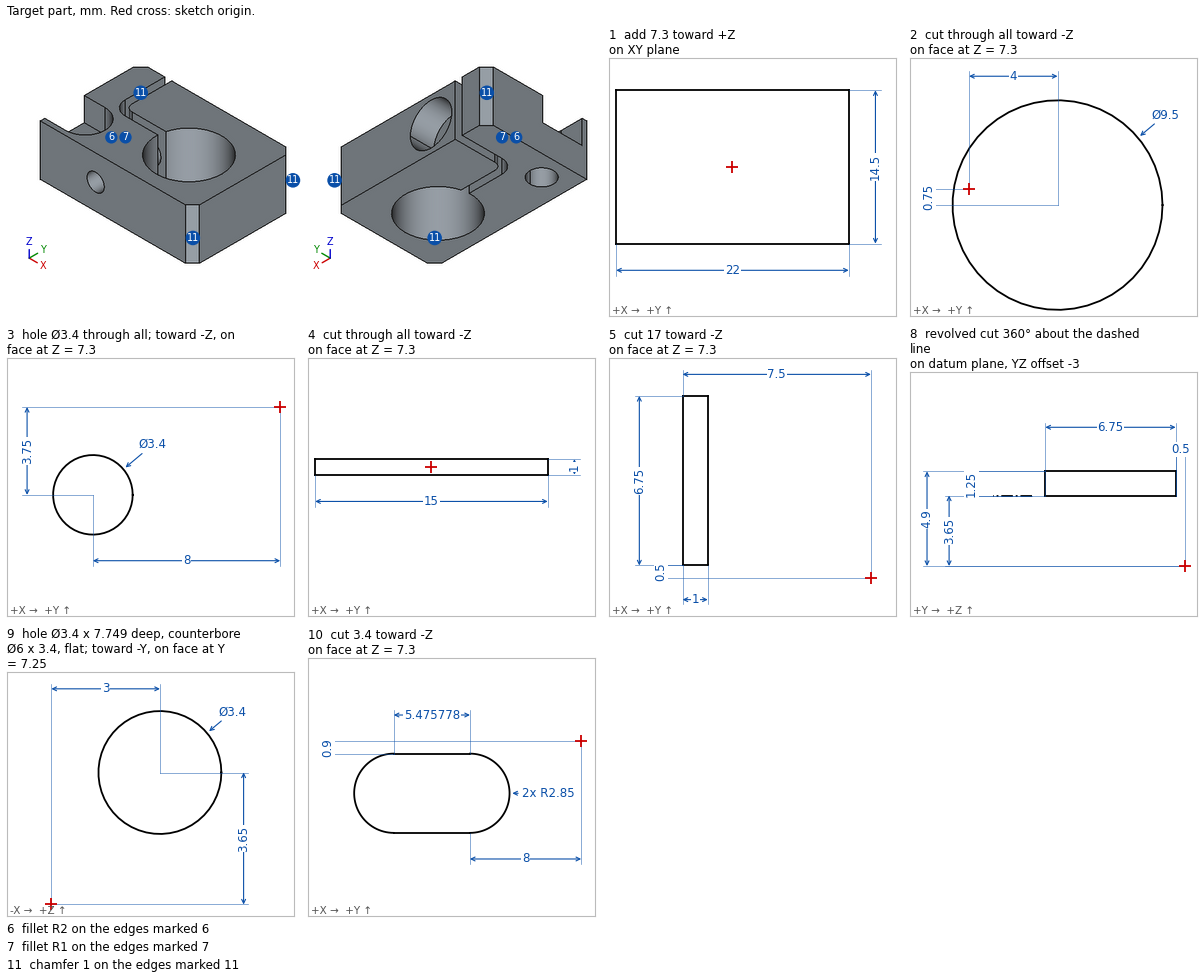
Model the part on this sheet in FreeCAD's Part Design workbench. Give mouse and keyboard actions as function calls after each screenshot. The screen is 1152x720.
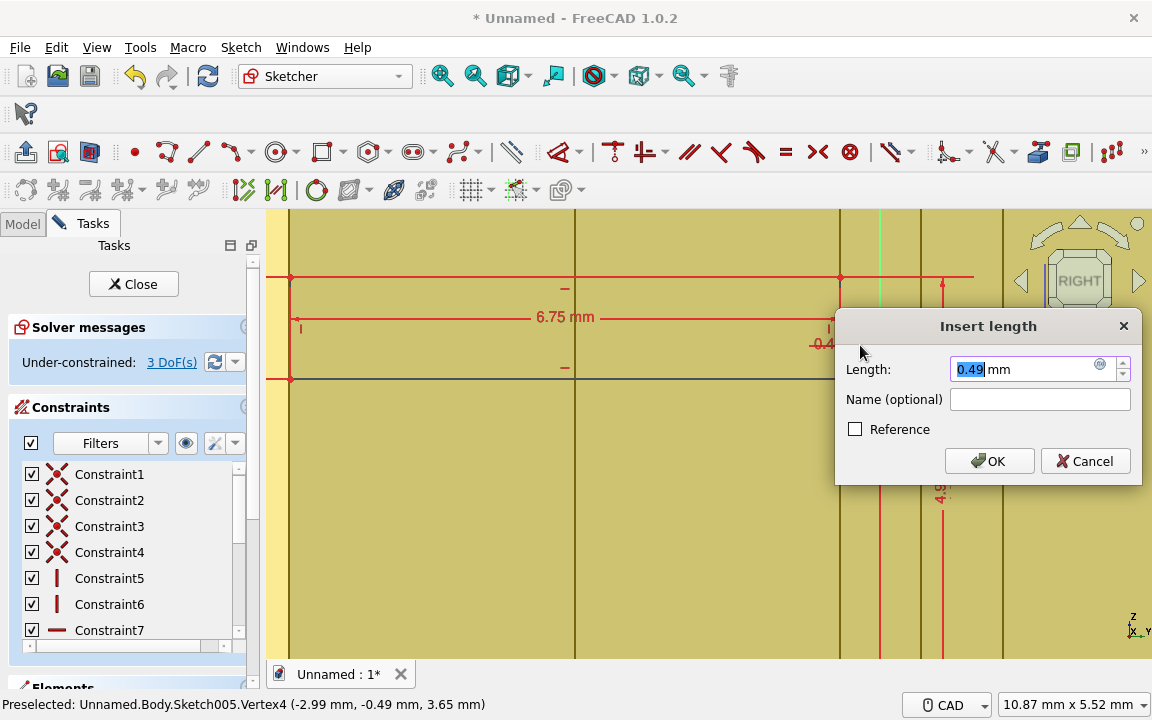
text(0.5)
key(Return)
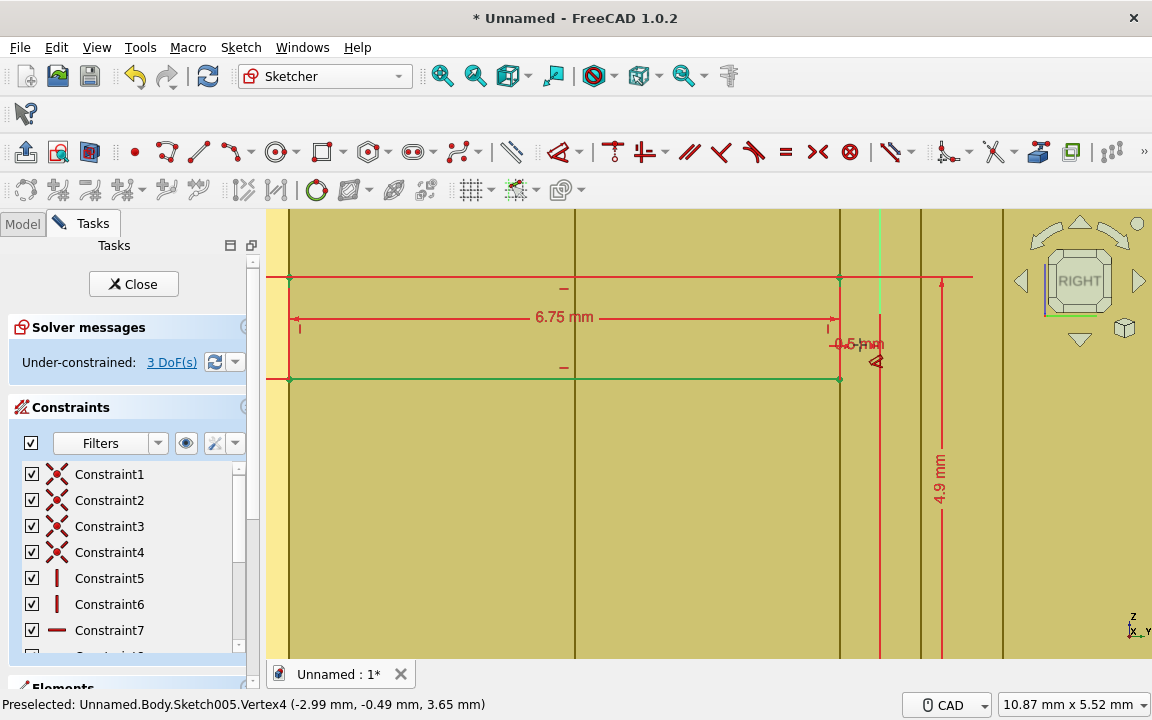
scroll(842, 382, down, 3)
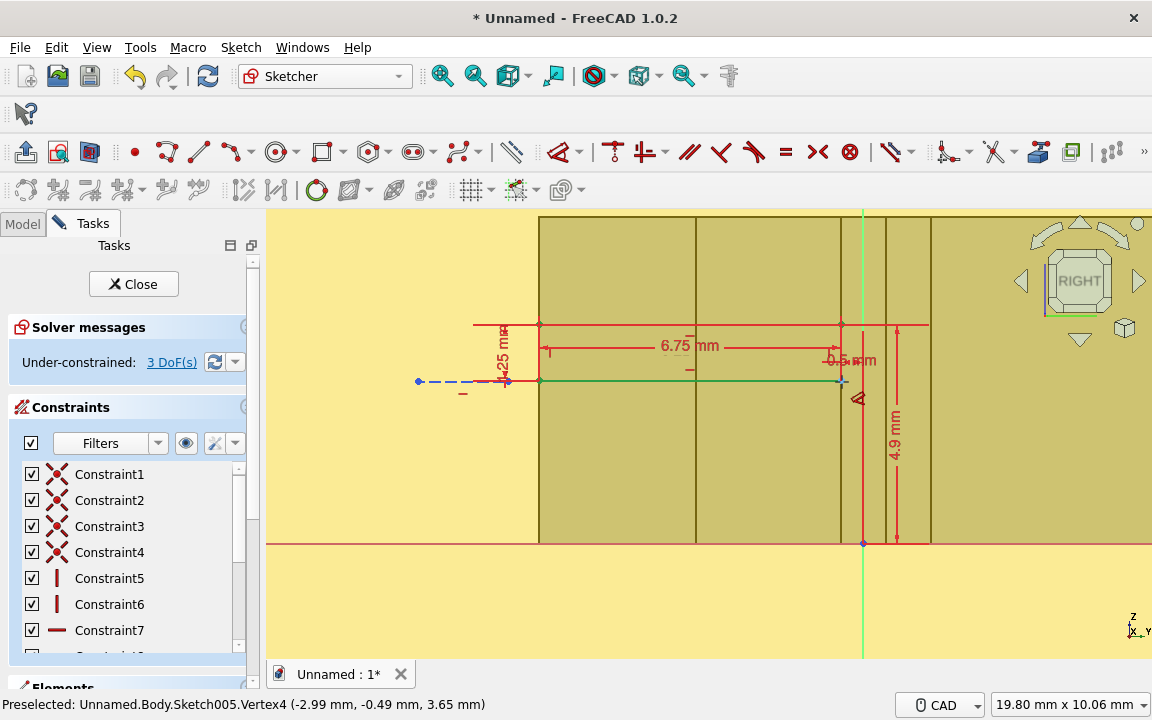
click(508, 382)
click(897, 463)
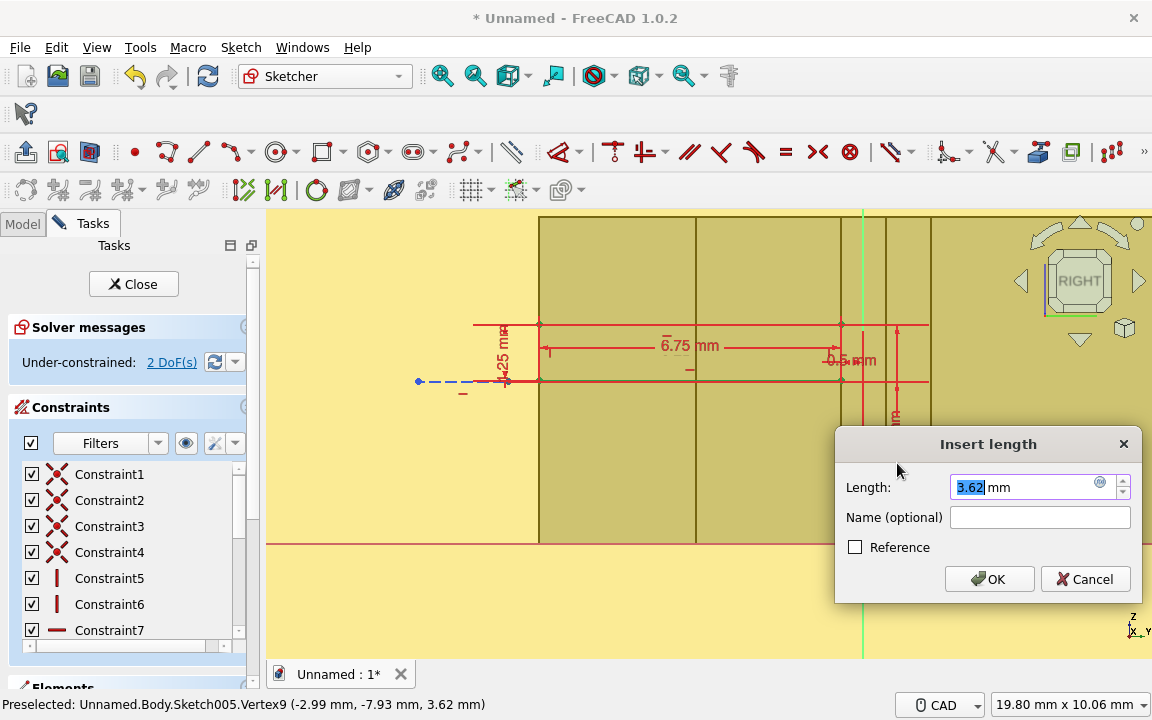
text(3.65)
key(Return)
key(Escape)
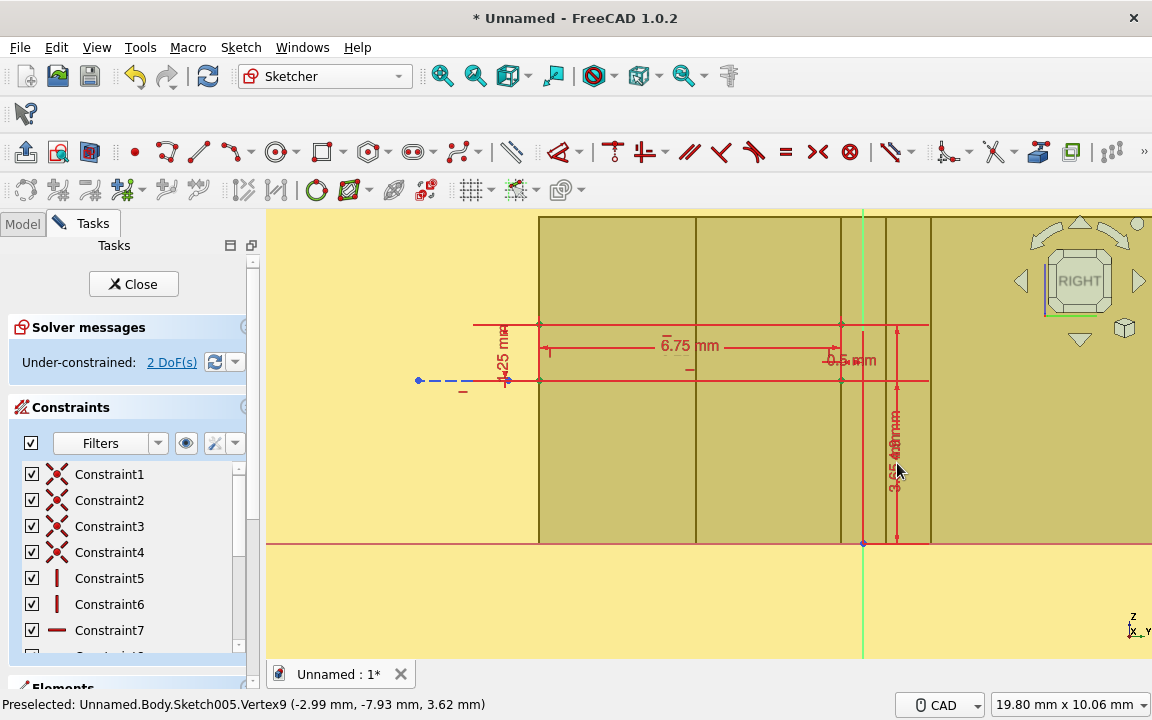
click(134, 284)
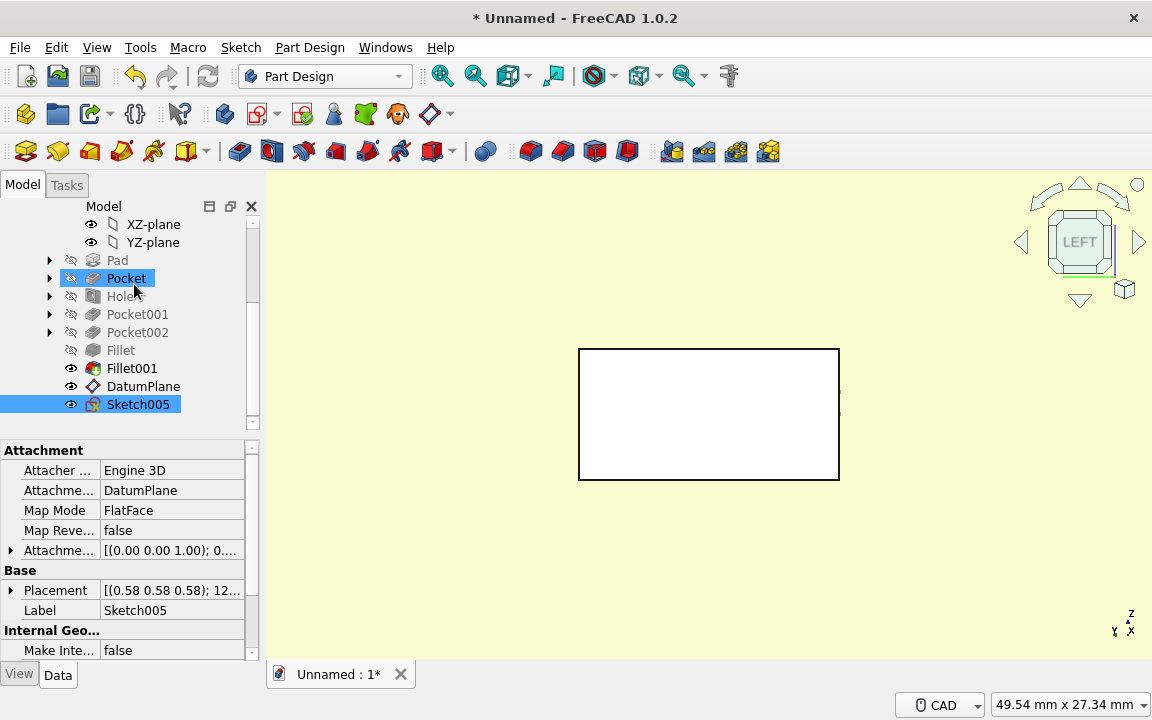
click(304, 152)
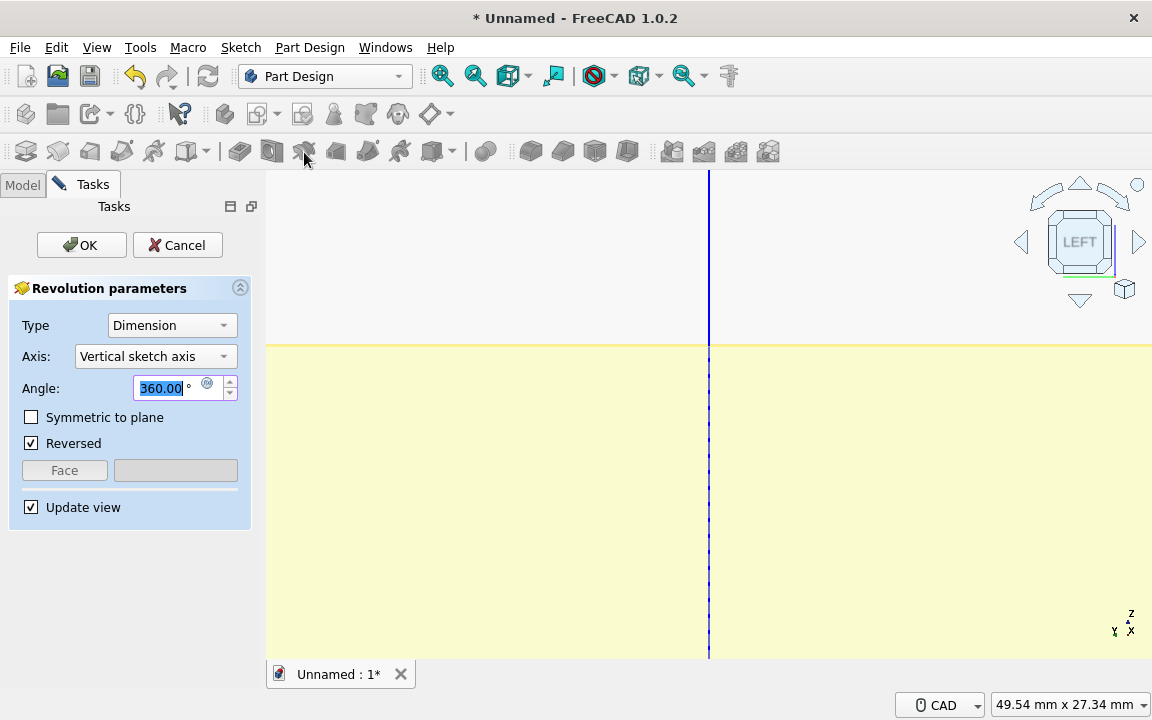
click(156, 356)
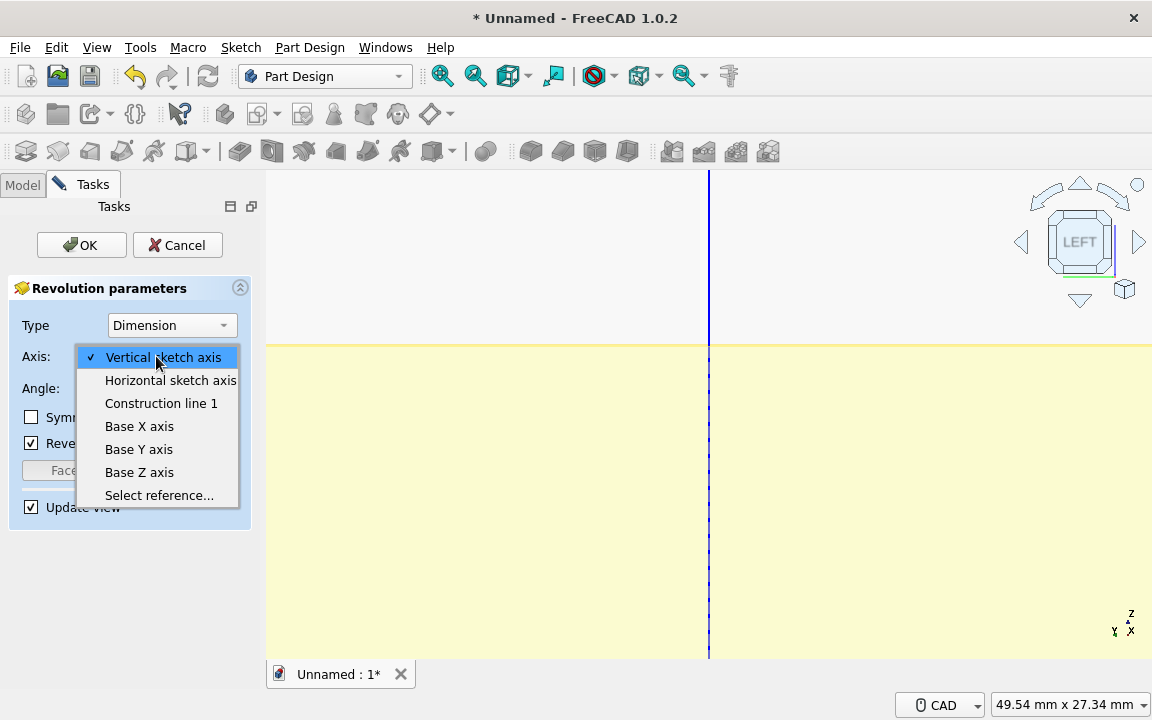
click(156, 404)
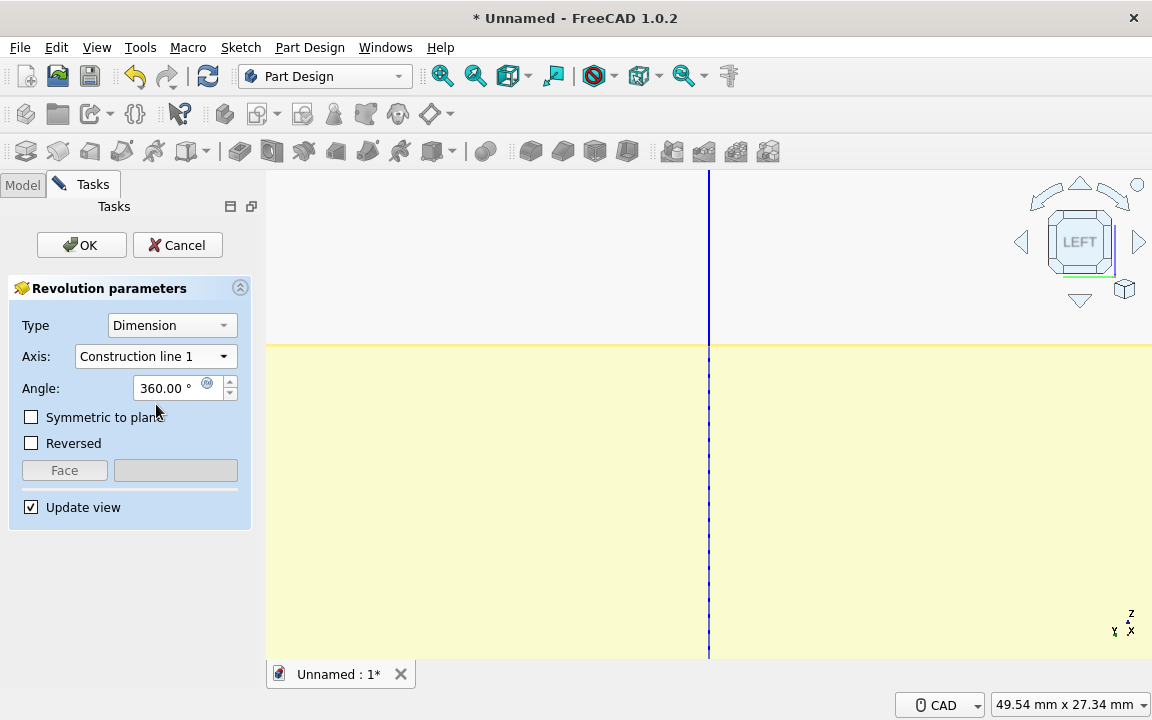
click(82, 245)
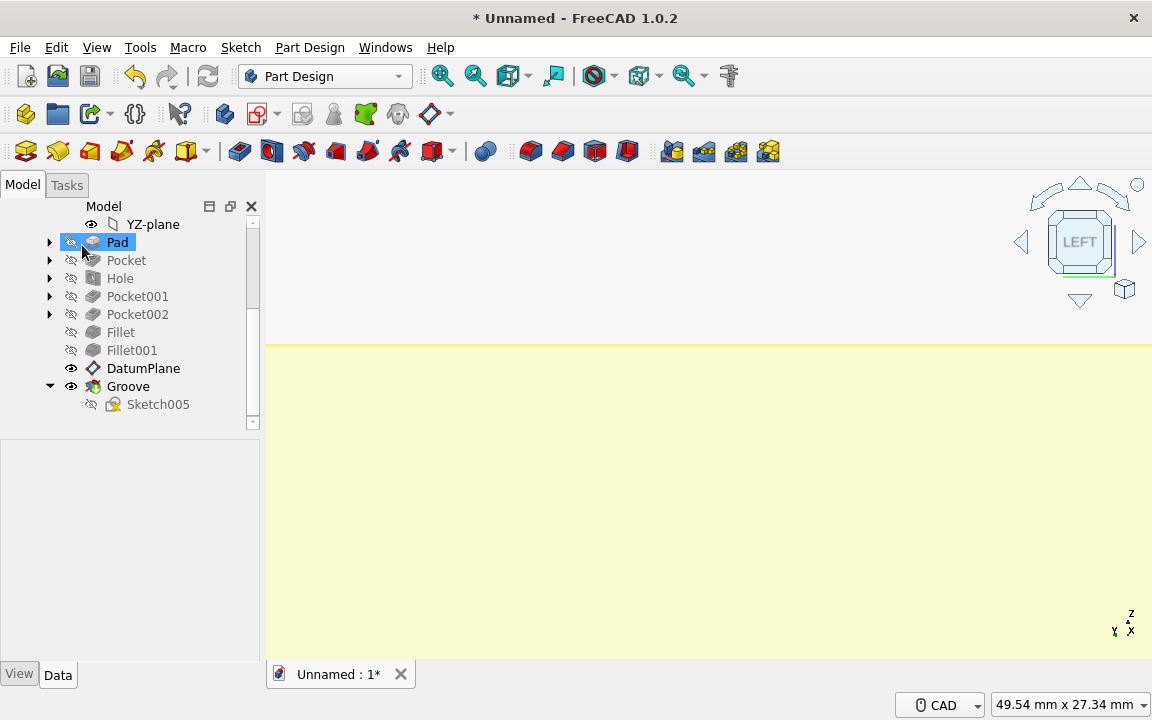
click(116, 368)
key(space)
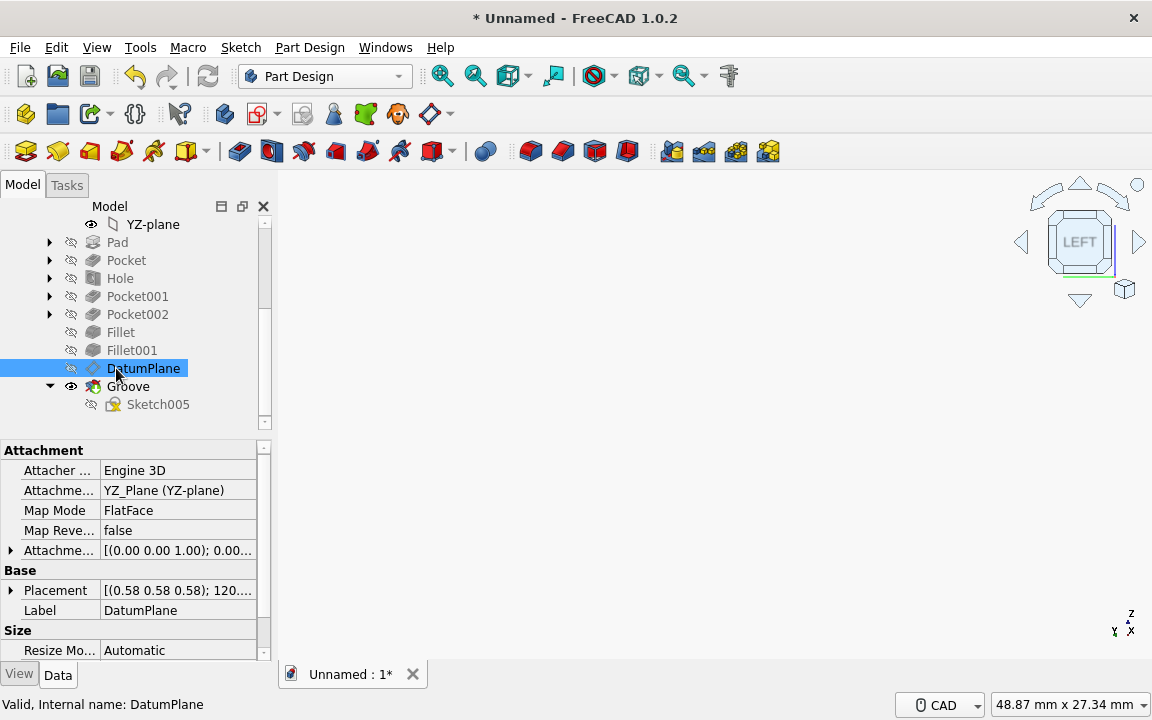
key(v)
key(f)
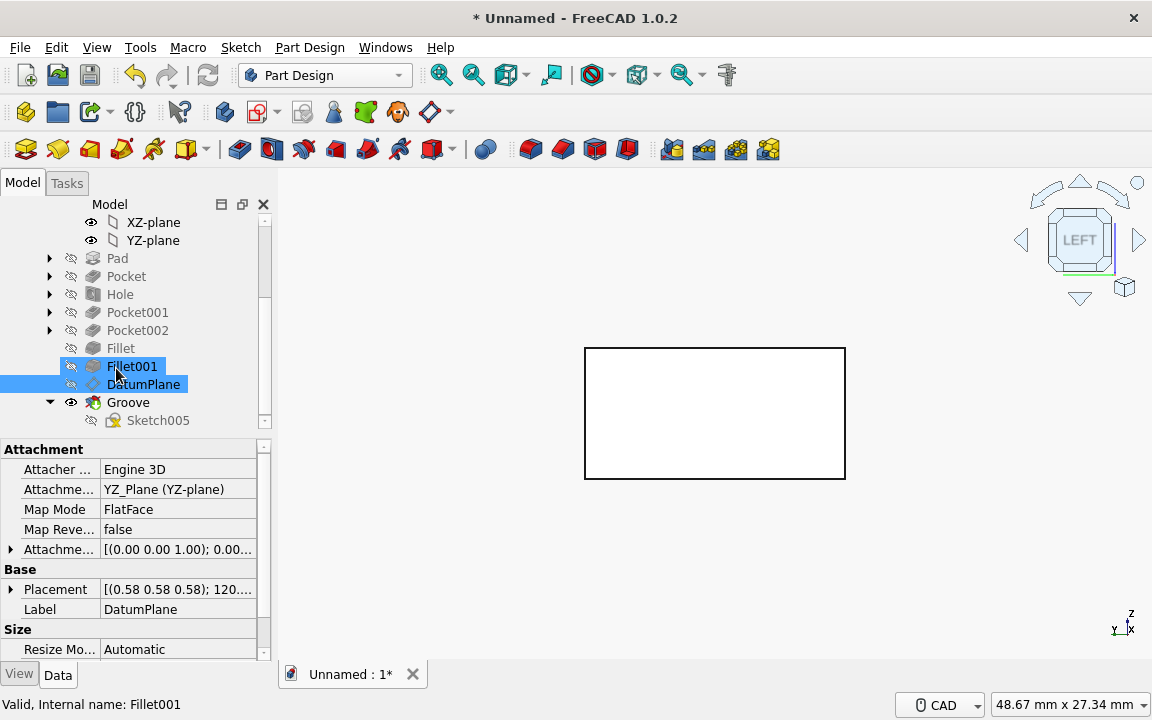
key(4)